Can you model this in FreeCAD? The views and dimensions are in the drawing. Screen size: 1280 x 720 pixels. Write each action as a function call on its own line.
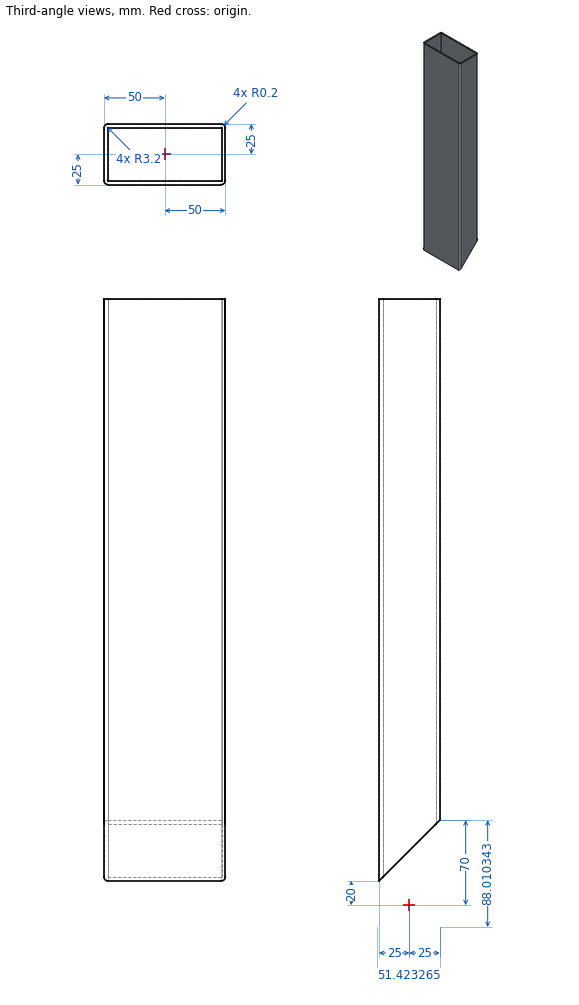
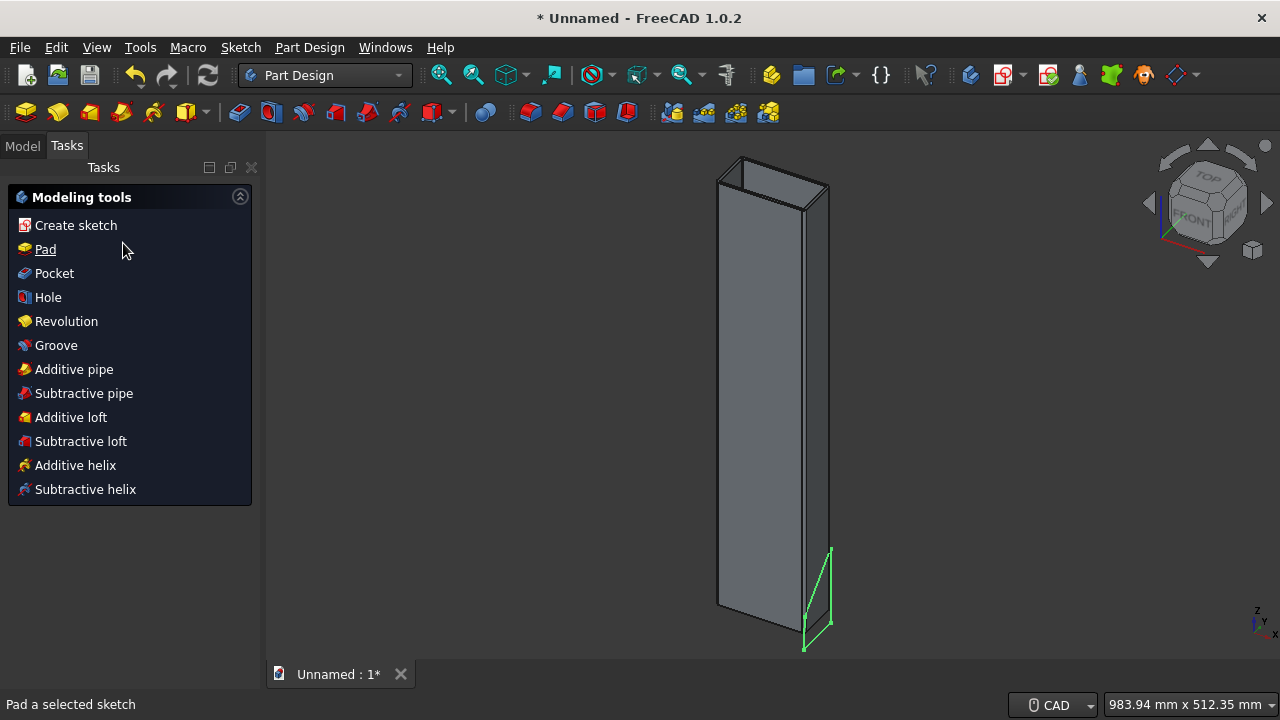
click(240, 112)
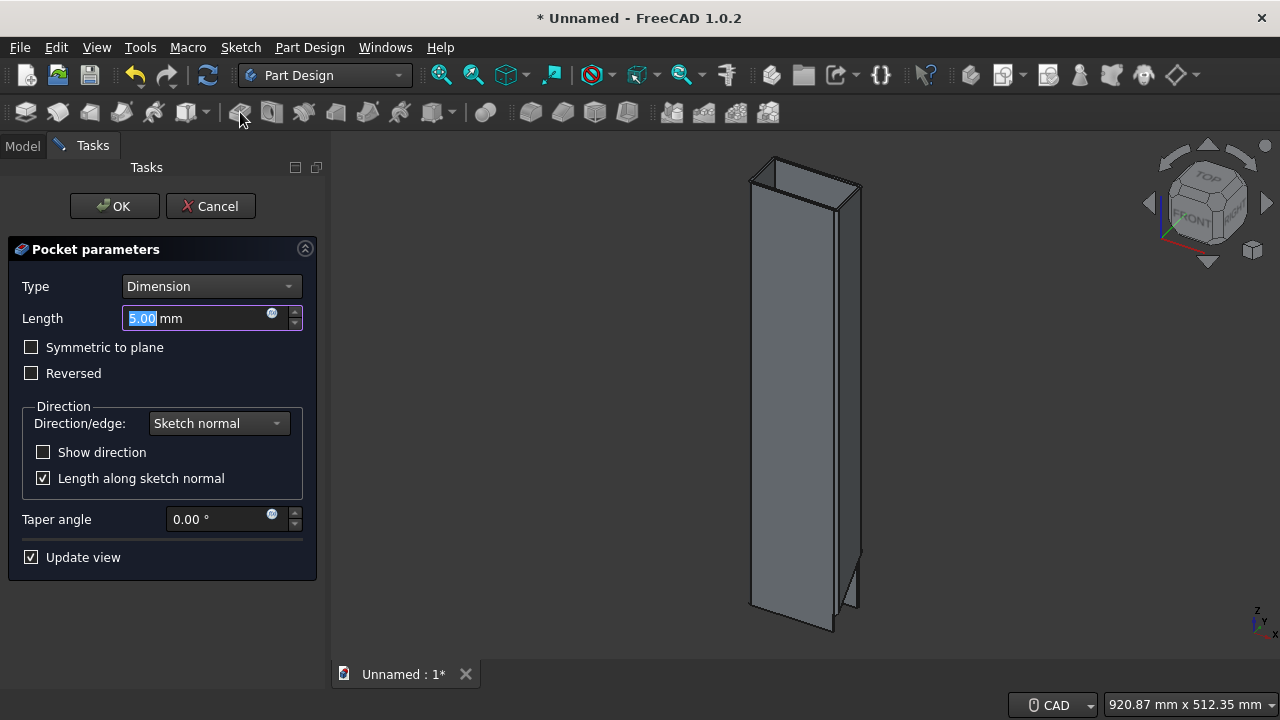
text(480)
key(Tab)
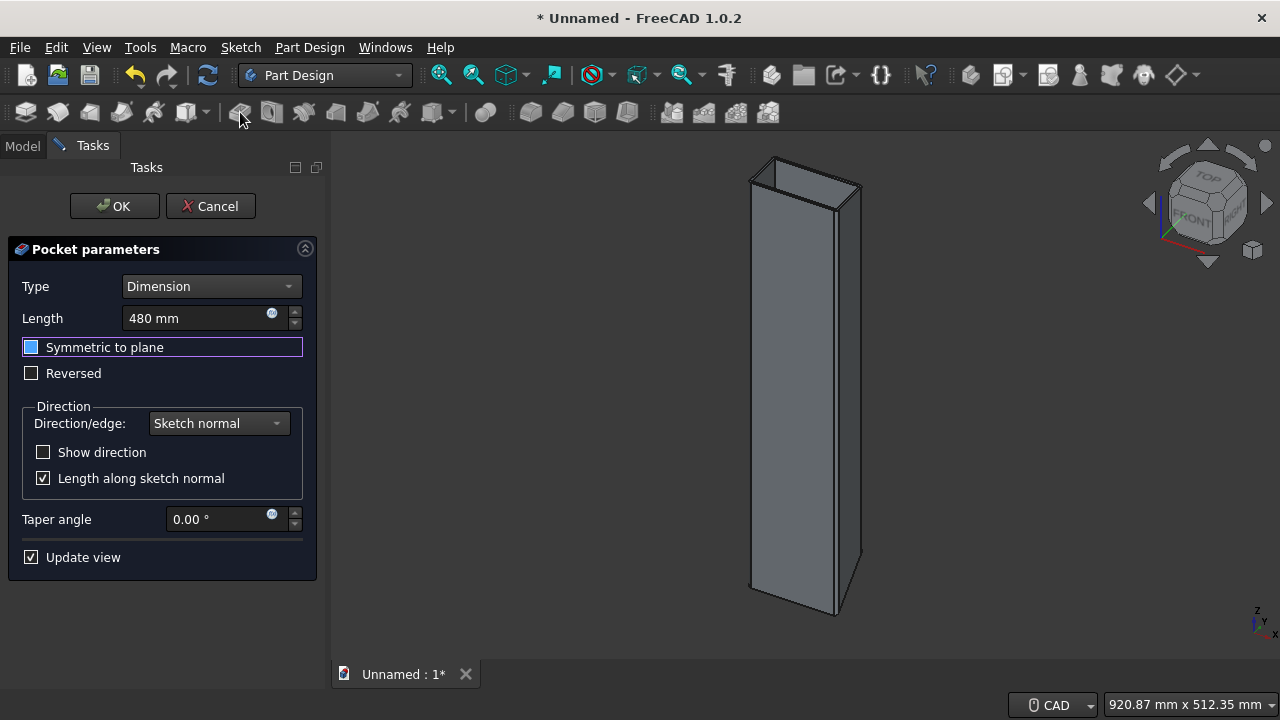
click(115, 206)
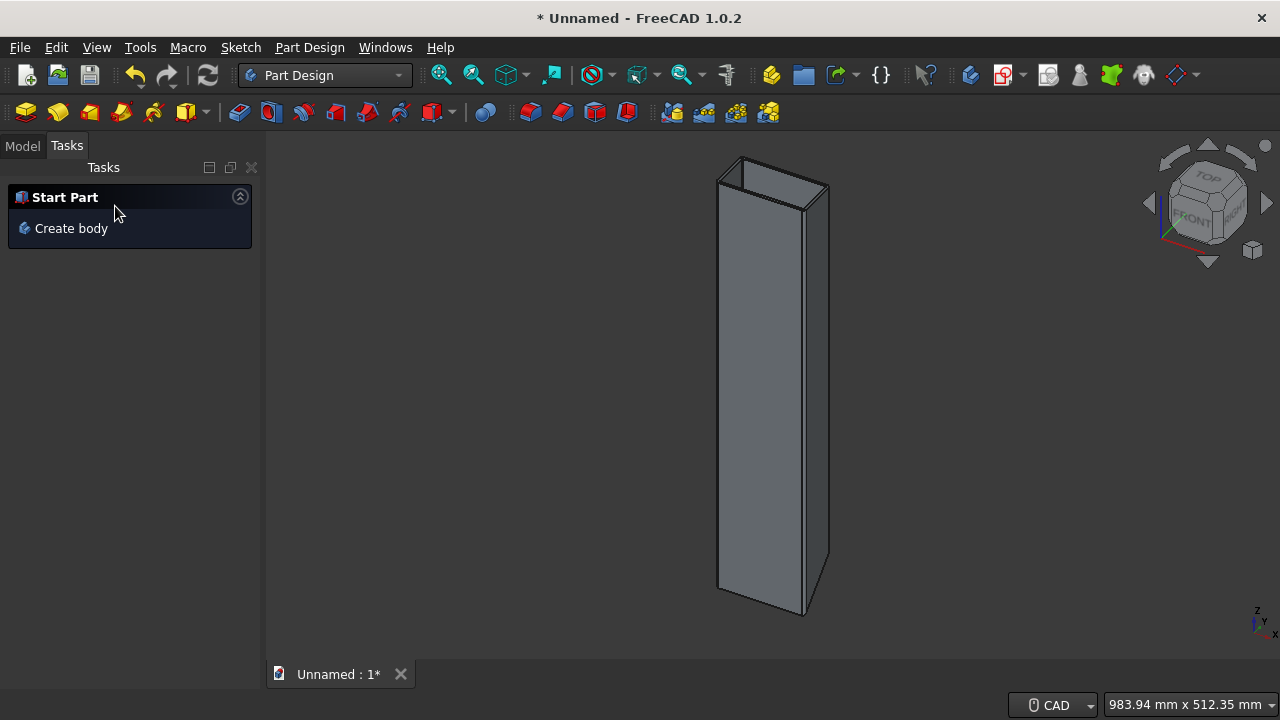
key(0)